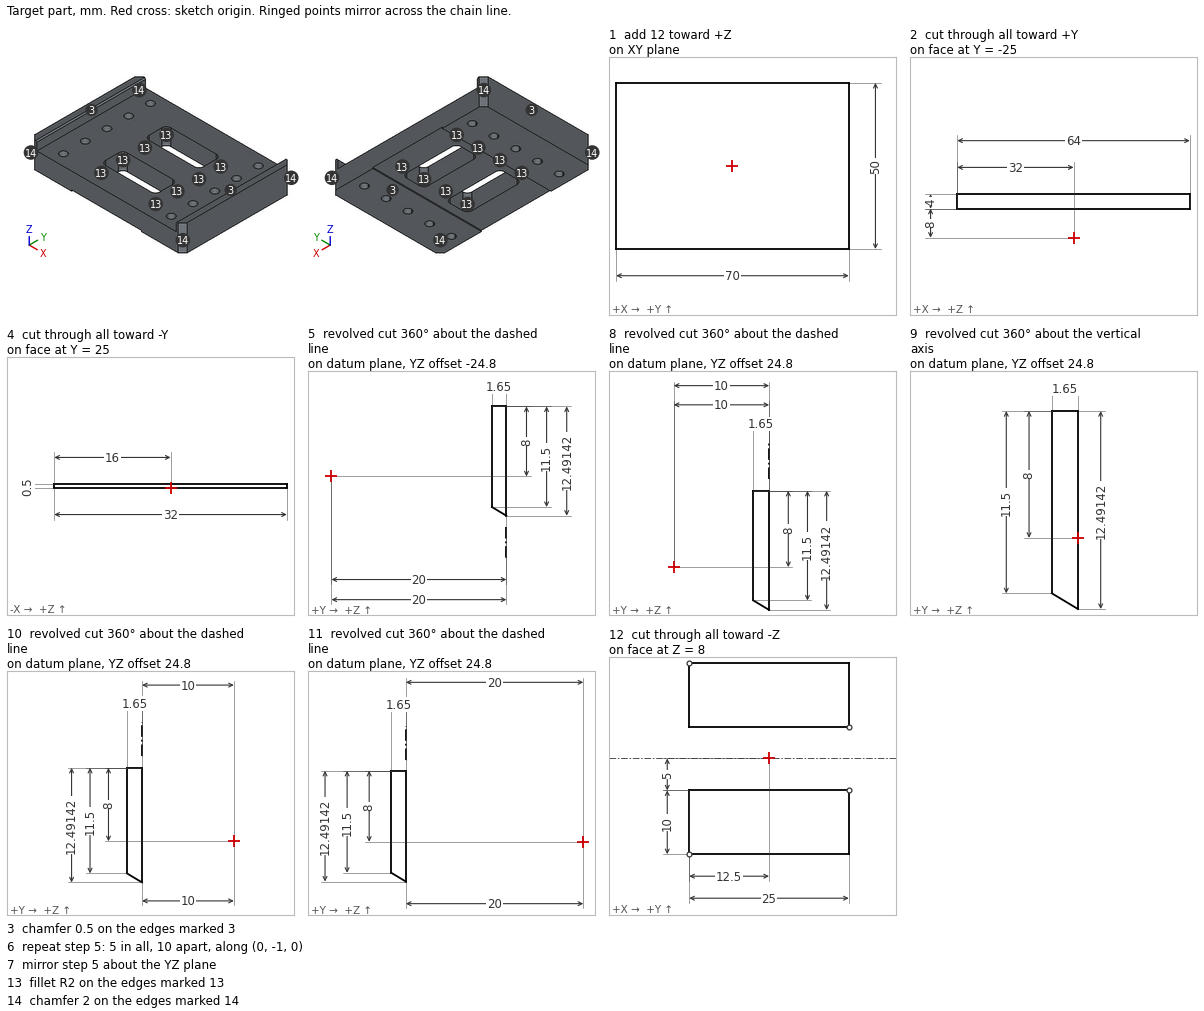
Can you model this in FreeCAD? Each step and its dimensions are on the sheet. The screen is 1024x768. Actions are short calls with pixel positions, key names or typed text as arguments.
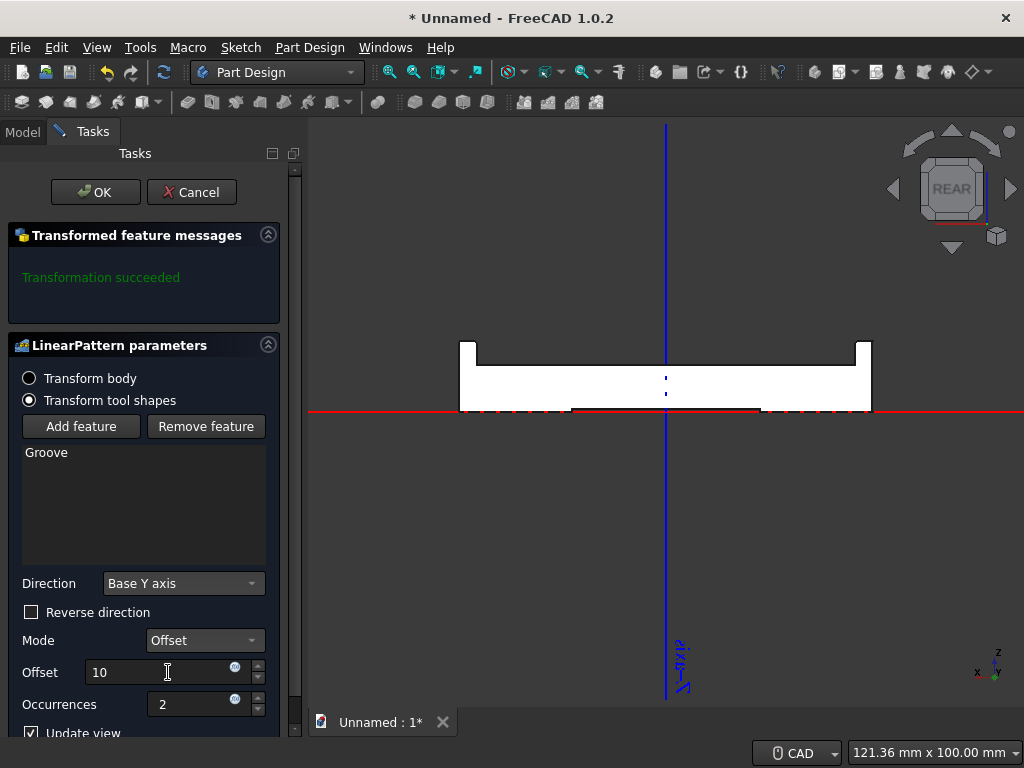
triple_click(198, 704)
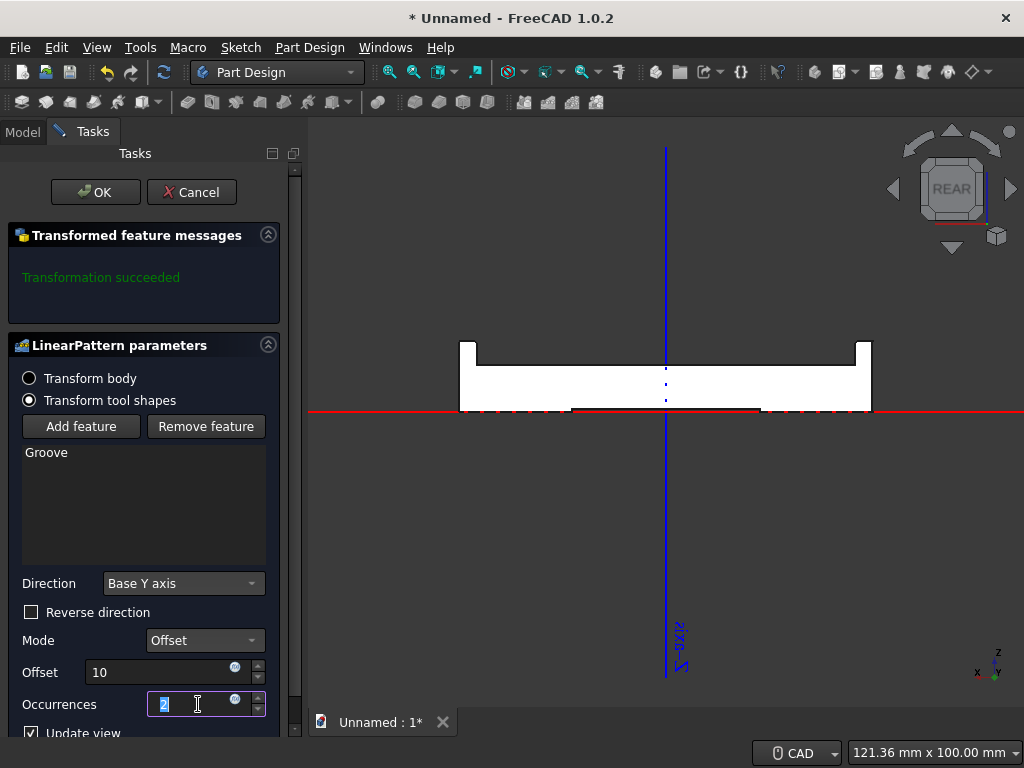
text(5)
key(Tab)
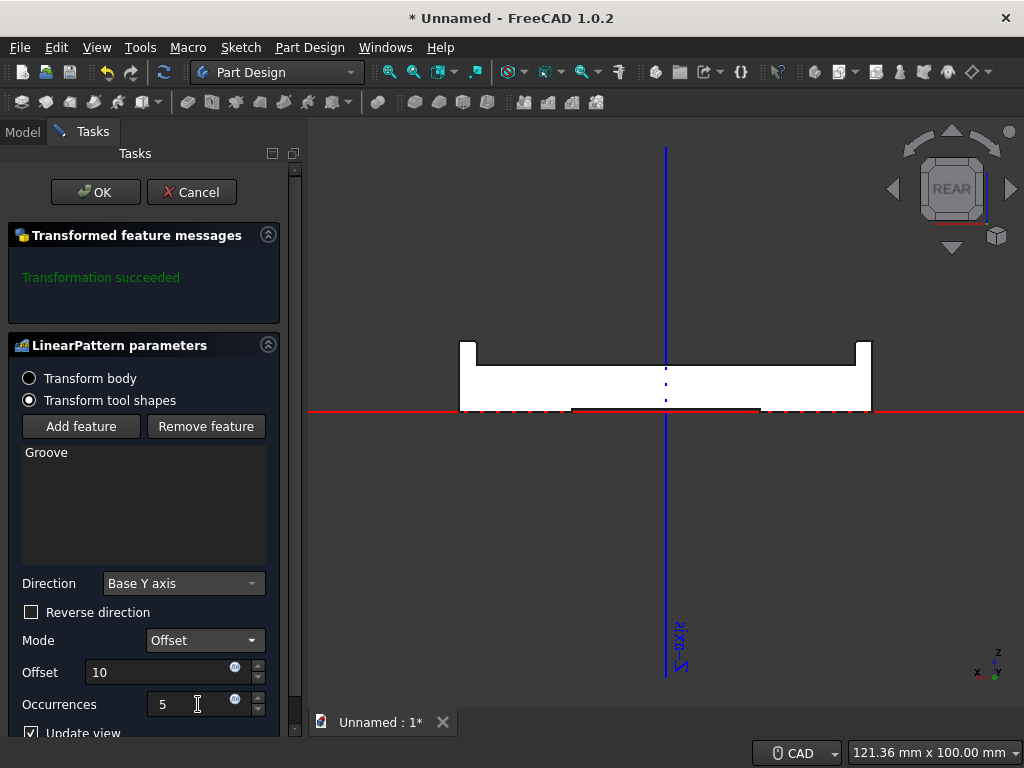
click(30, 612)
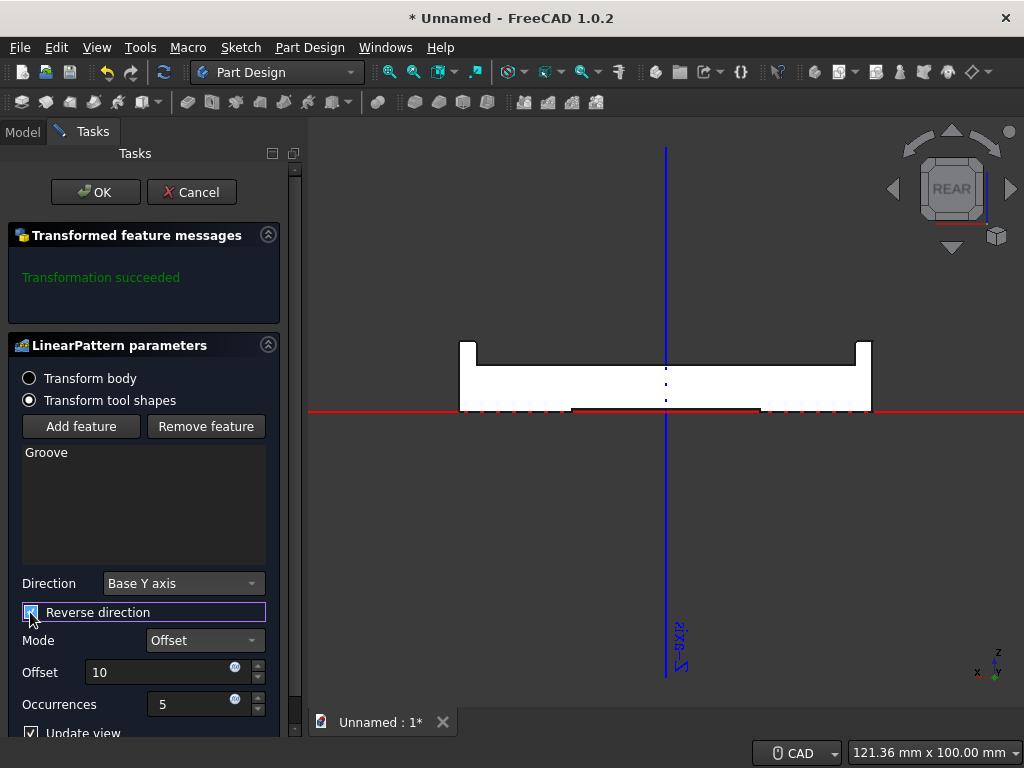
click(96, 192)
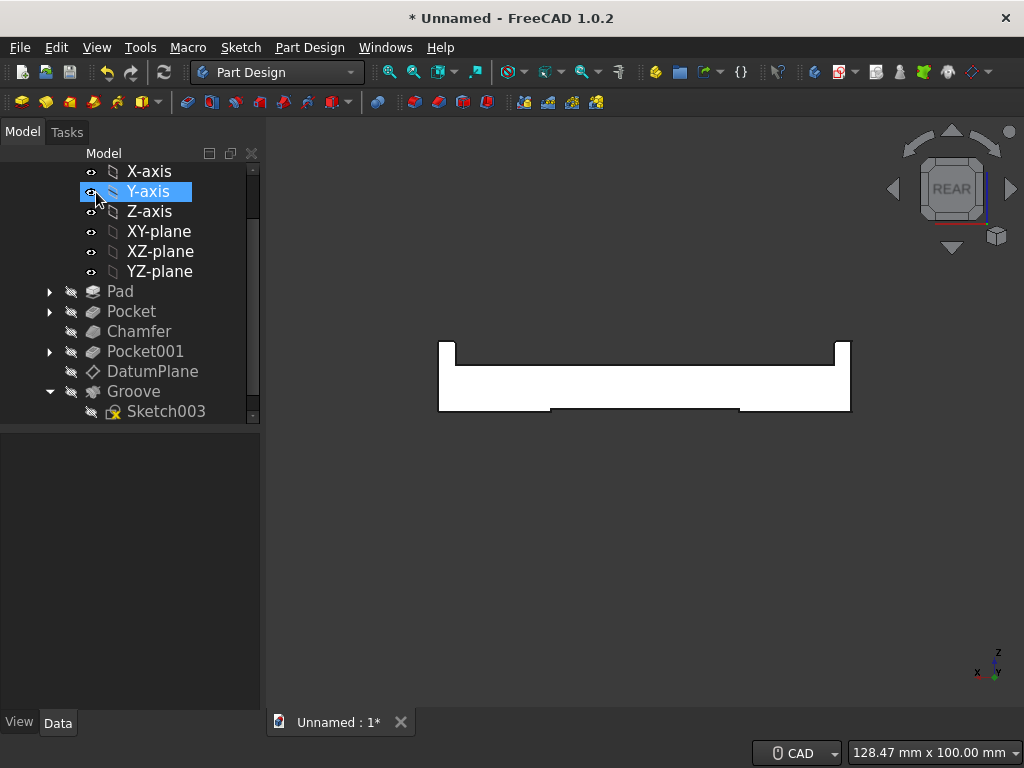
click(116, 392)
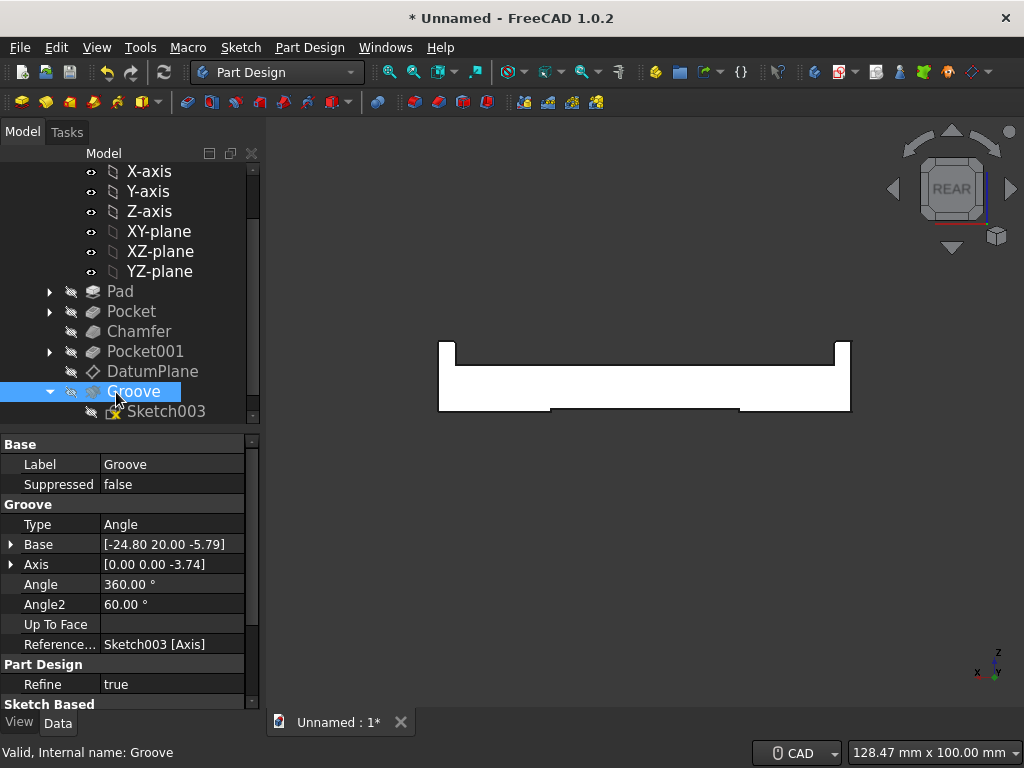
click(524, 102)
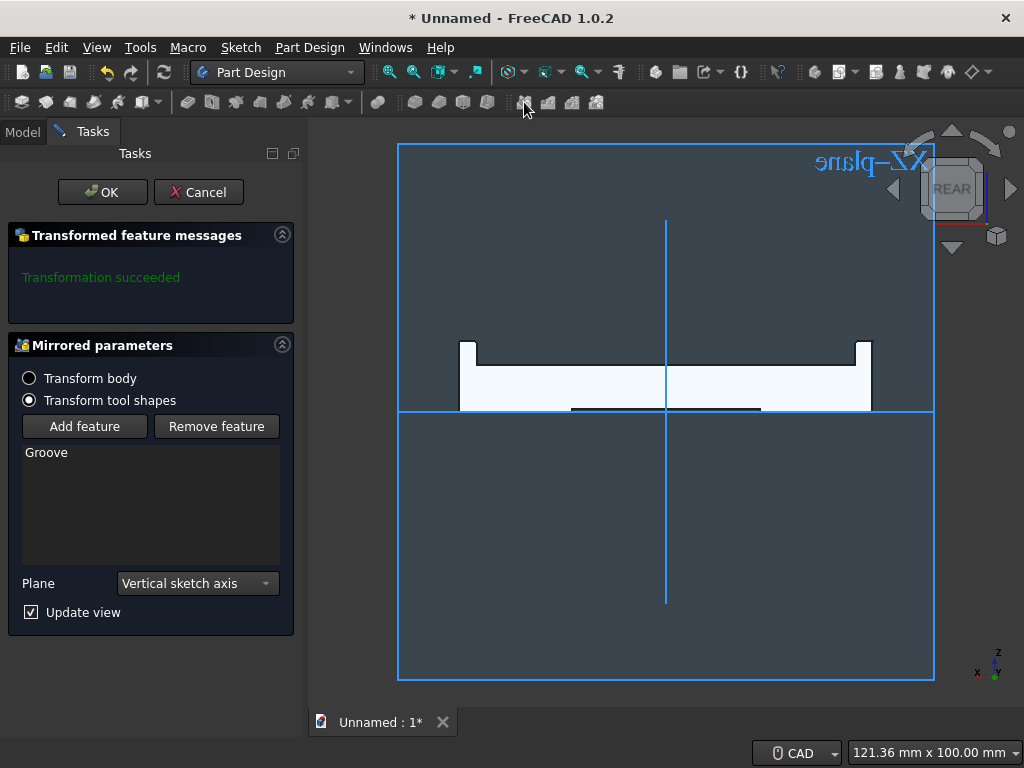
click(198, 584)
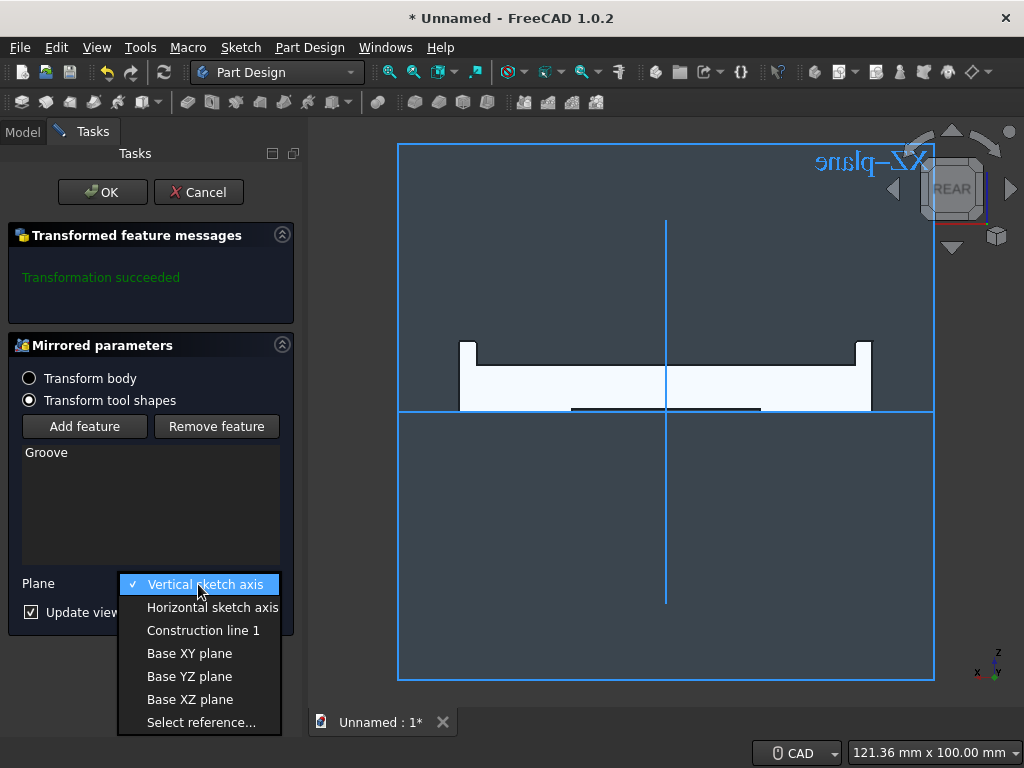
click(198, 676)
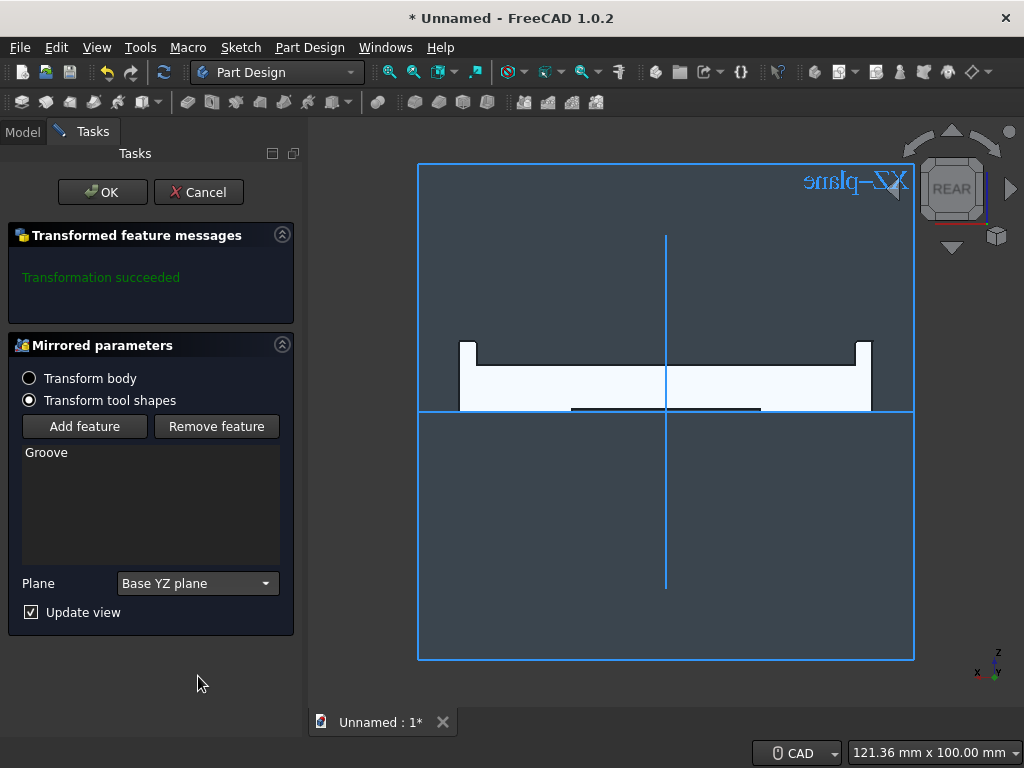
click(103, 192)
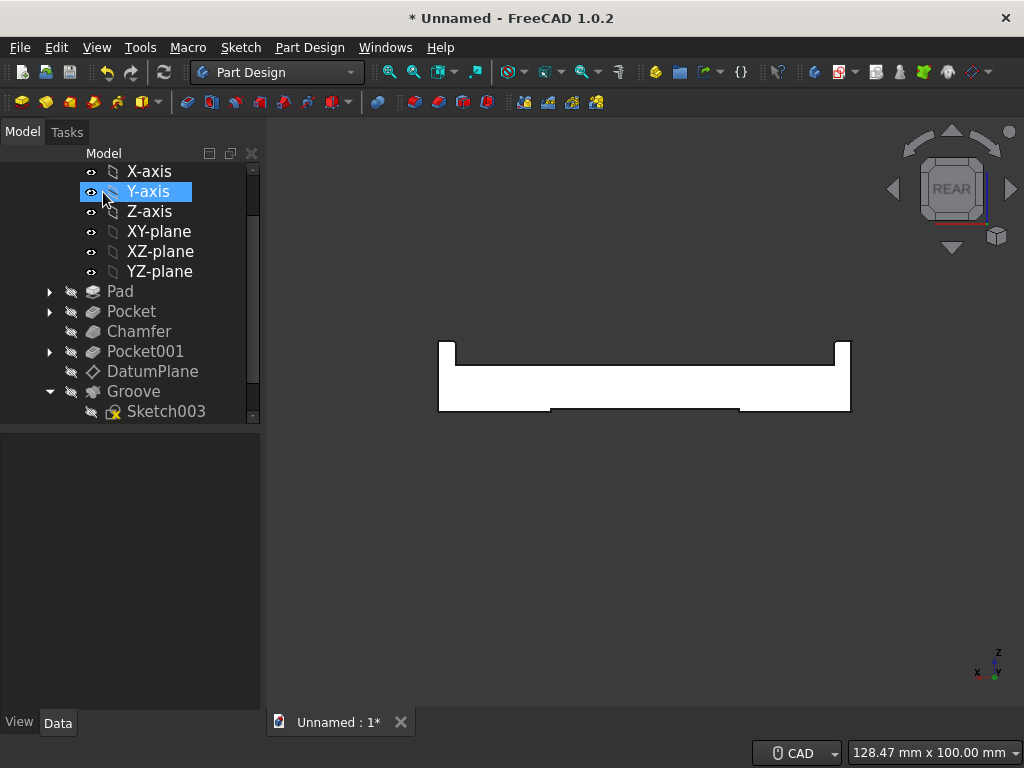
scroll(160, 287, down, 3)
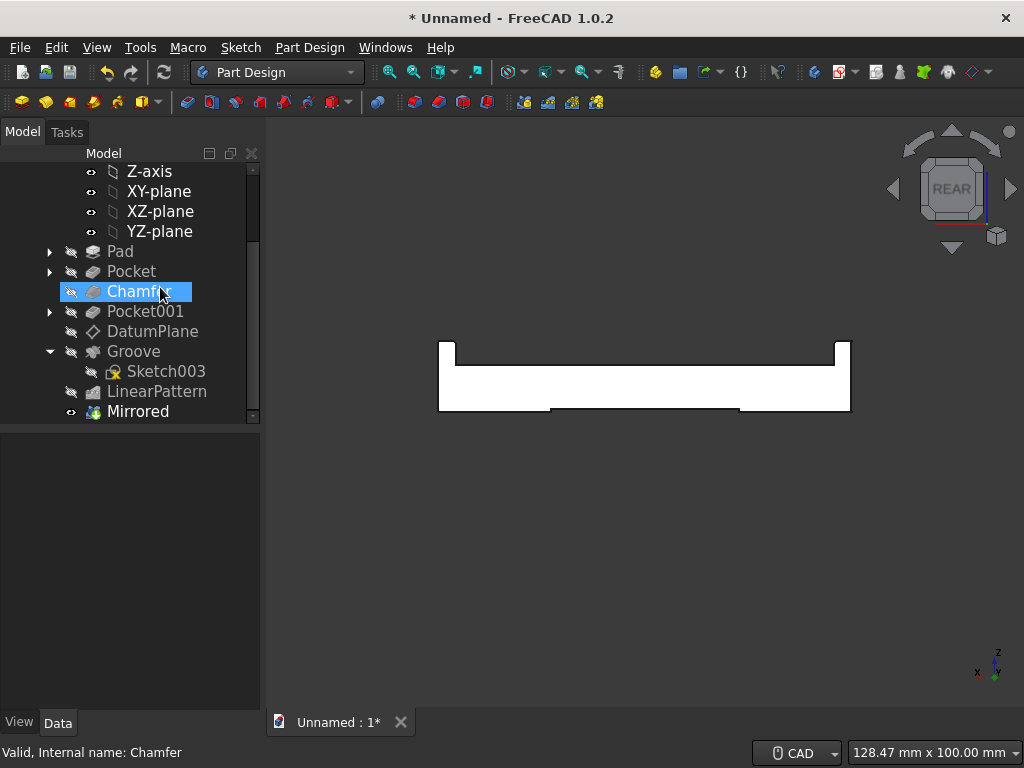
scroll(160, 287, up, 15)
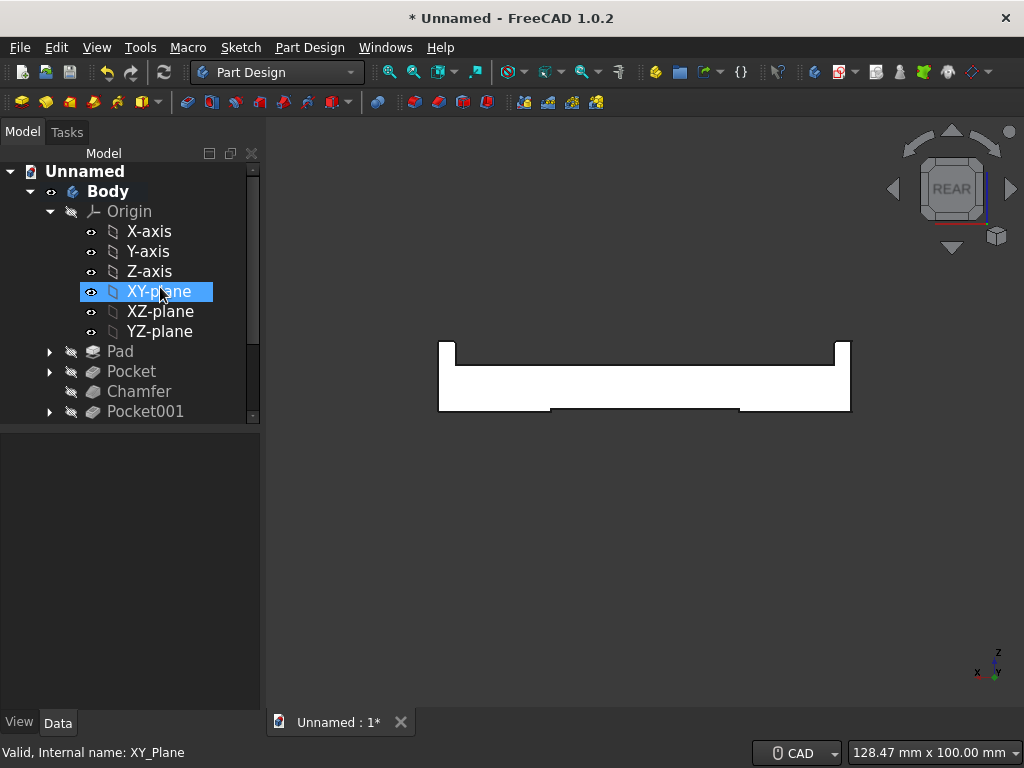
click(136, 332)